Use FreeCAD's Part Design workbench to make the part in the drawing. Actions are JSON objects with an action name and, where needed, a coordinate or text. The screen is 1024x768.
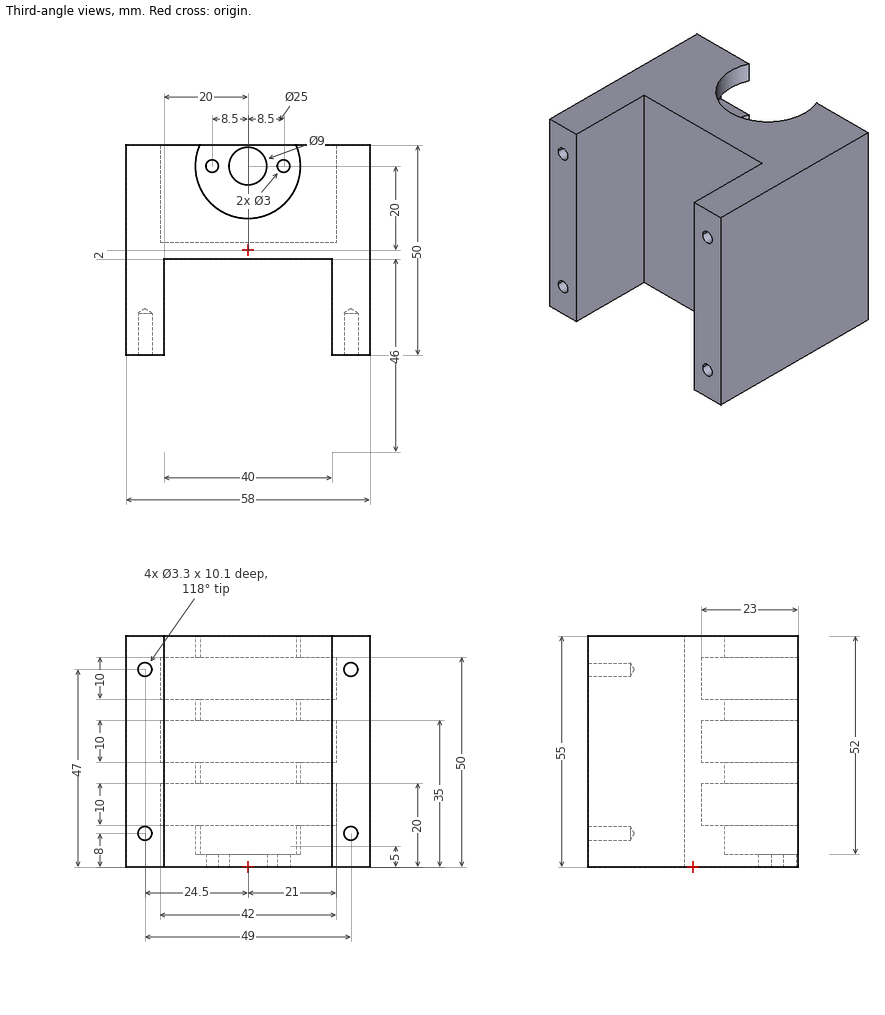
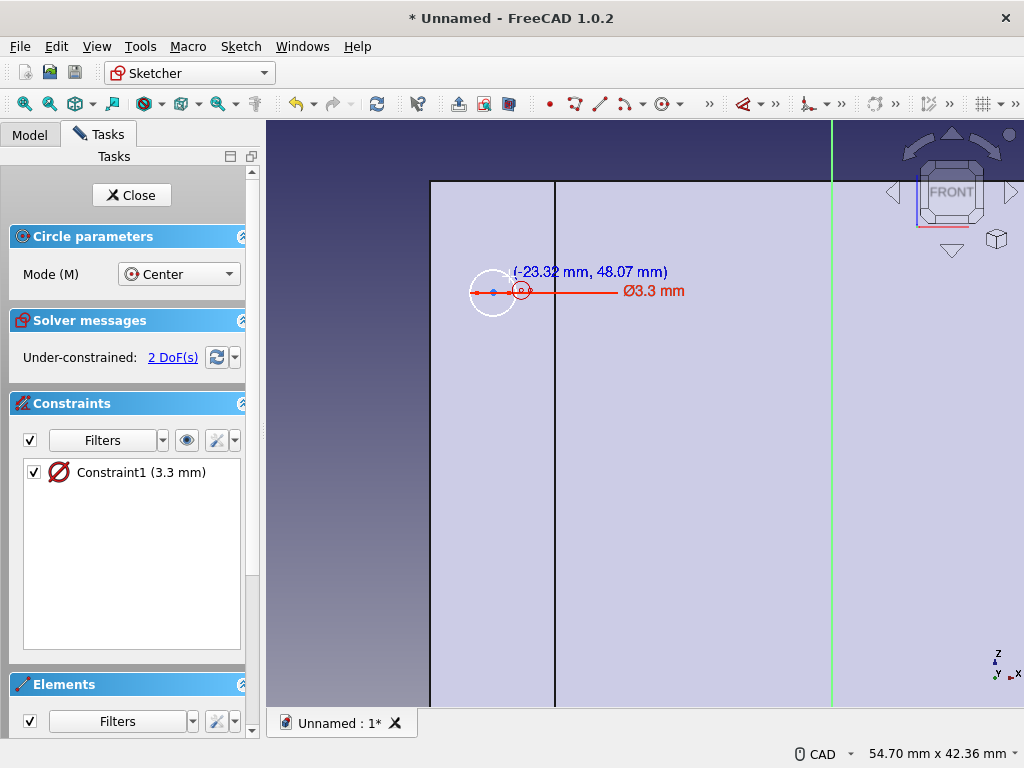
{"action": "scroll", "coordinate": [294, 179], "scroll_direction": "down", "scroll_amount": 3}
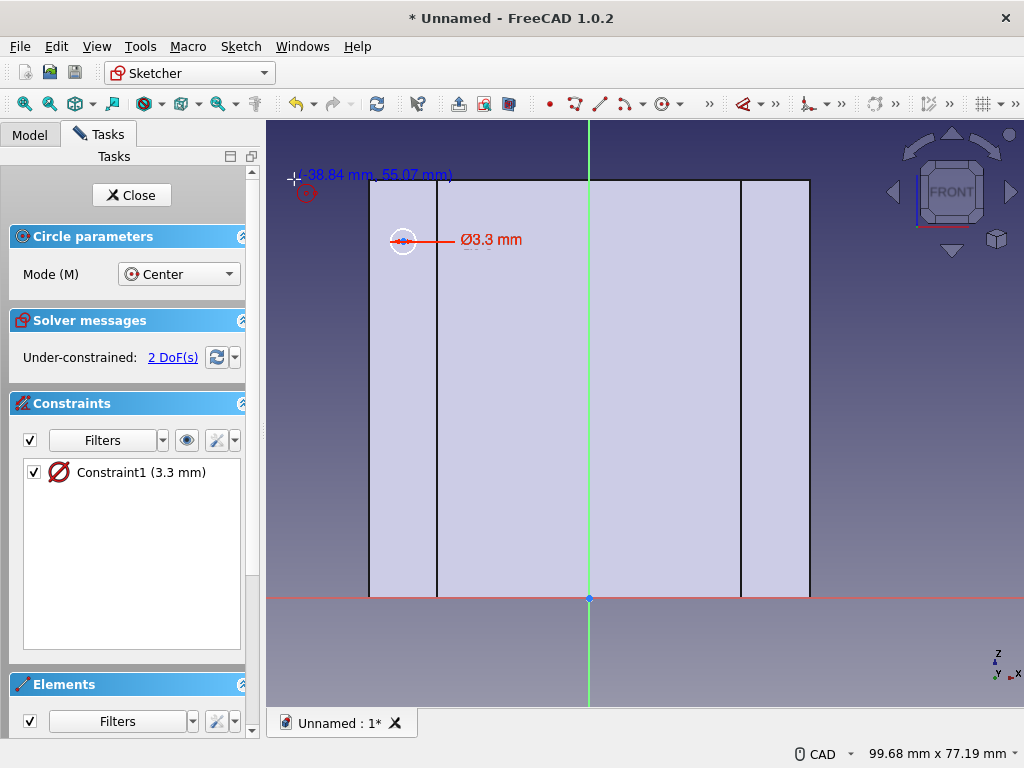
{"action": "scroll", "coordinate": [403, 538], "scroll_direction": "up", "scroll_amount": 3}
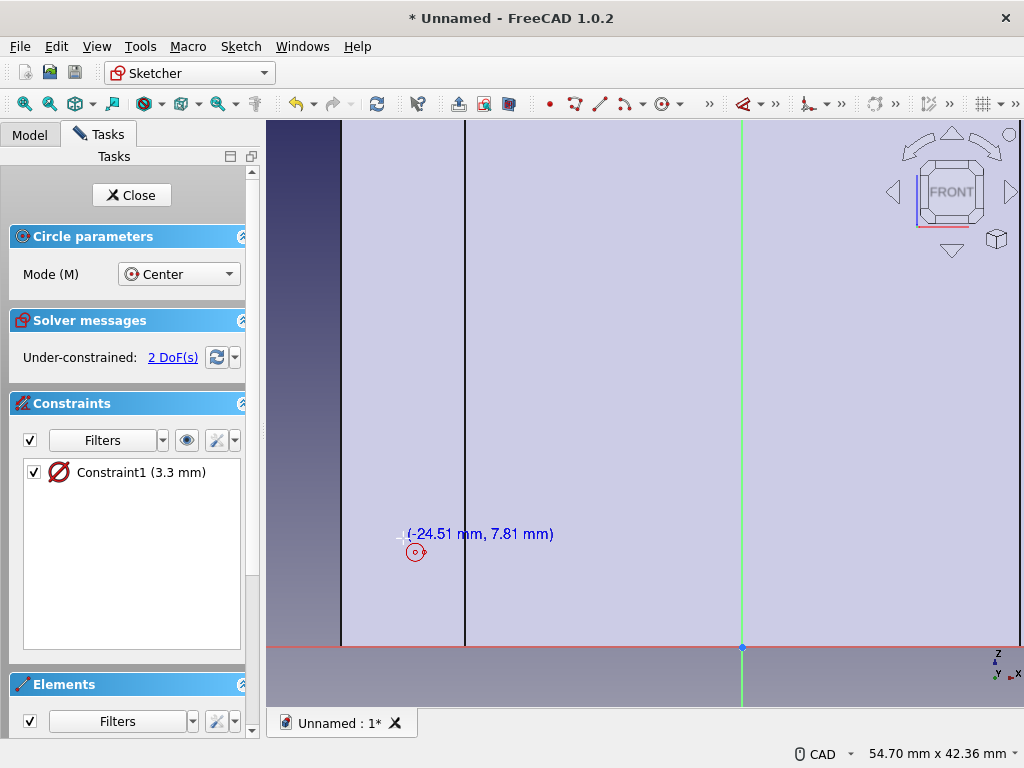
{"action": "left_click", "coordinate": [403, 537]}
{"action": "mouse_move", "coordinate": [419, 520]}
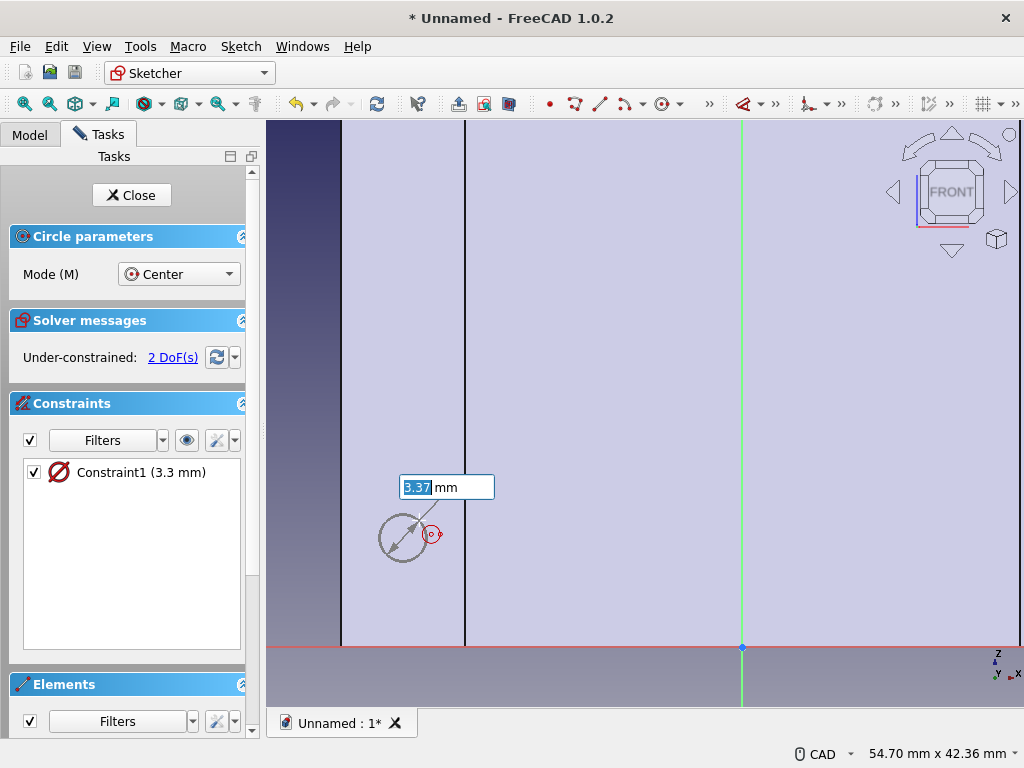
{"action": "type", "text": "3.3"}
{"action": "key", "text": "Return"}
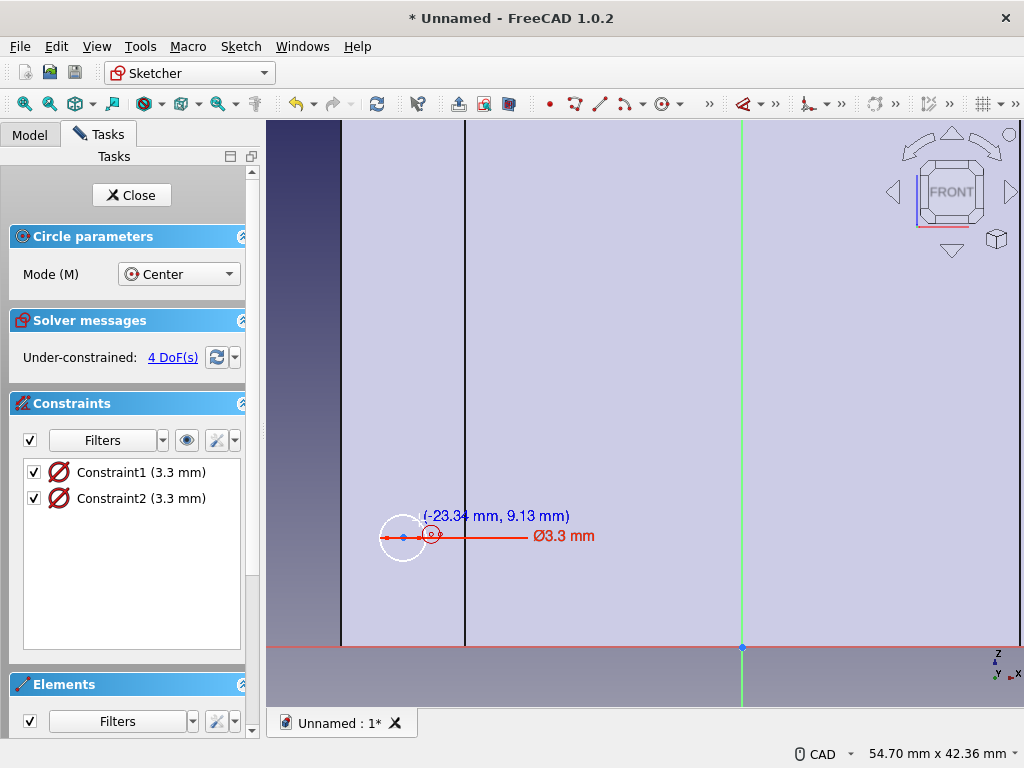
{"action": "scroll", "coordinate": [375, 539], "scroll_direction": "down", "scroll_amount": 3}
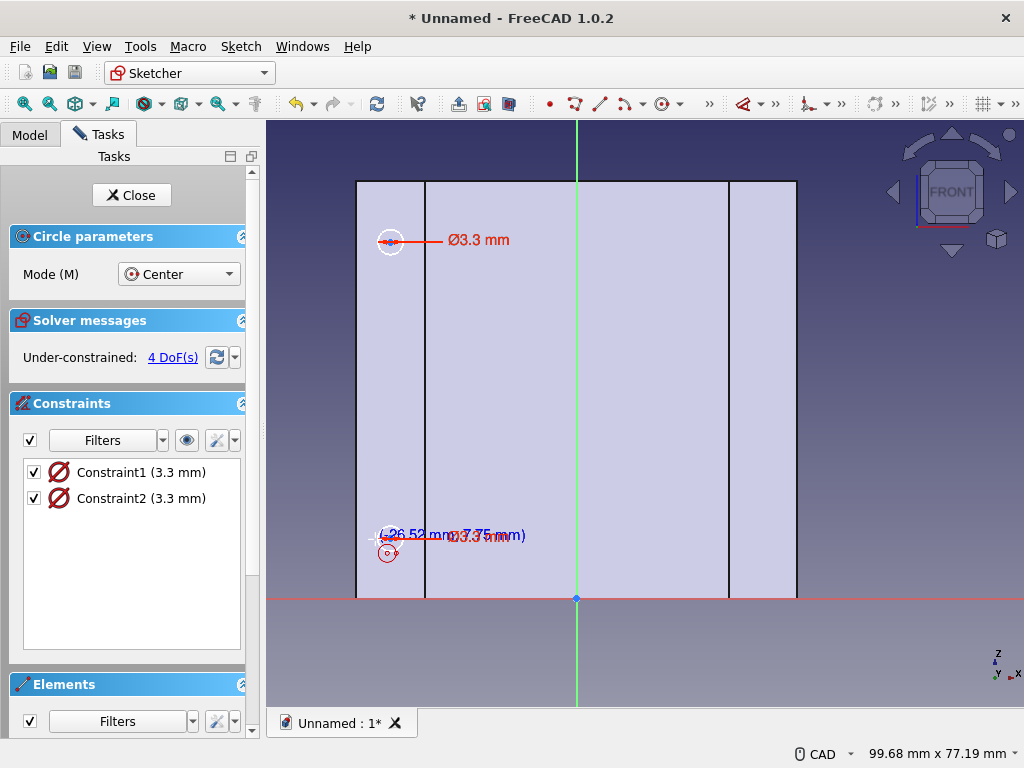
{"action": "scroll", "coordinate": [763, 538], "scroll_direction": "up", "scroll_amount": 3}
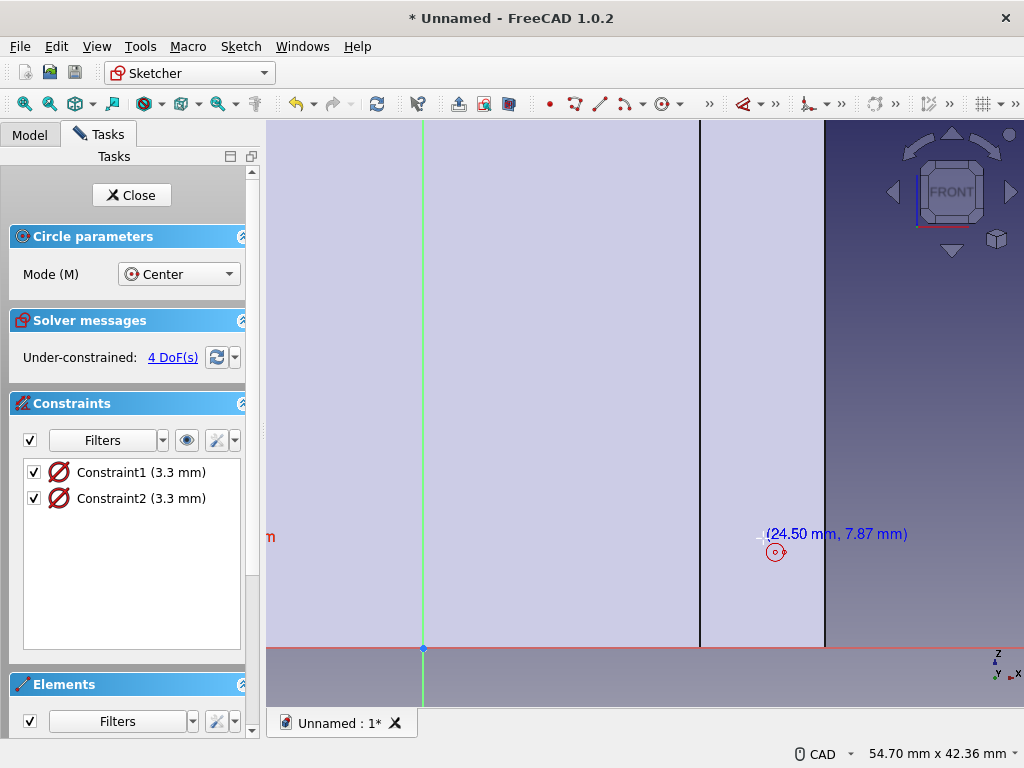
{"action": "left_click", "coordinate": [762, 537]}
{"action": "mouse_move", "coordinate": [779, 521]}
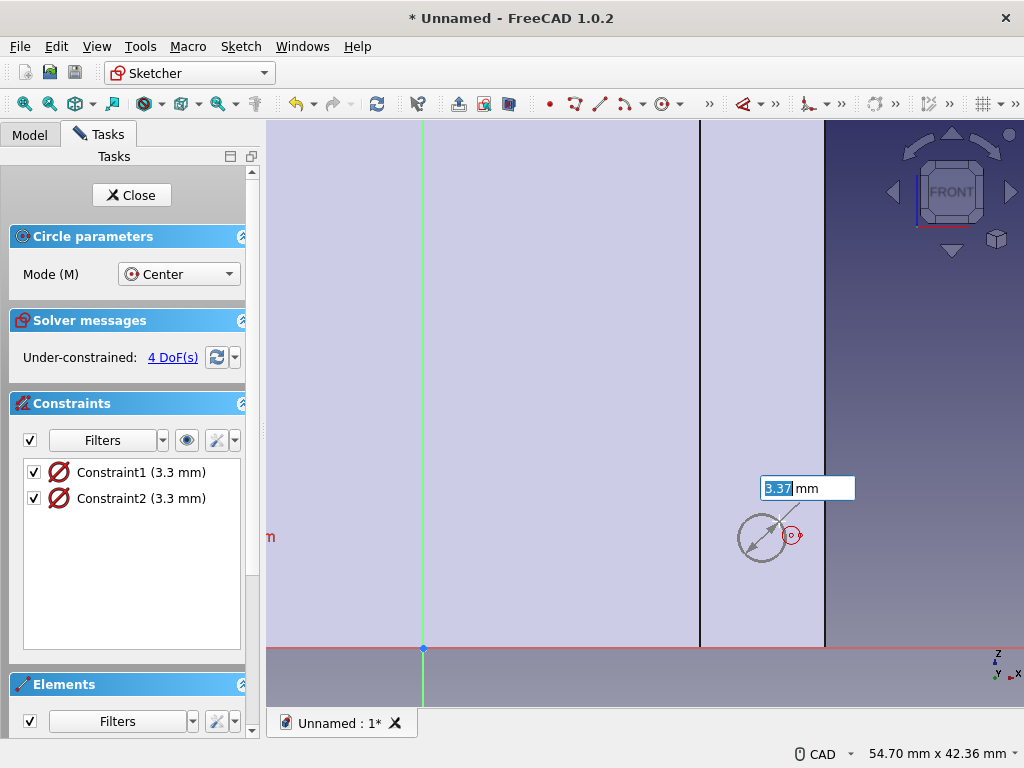
{"action": "type", "text": "3.3"}
{"action": "key", "text": "Return"}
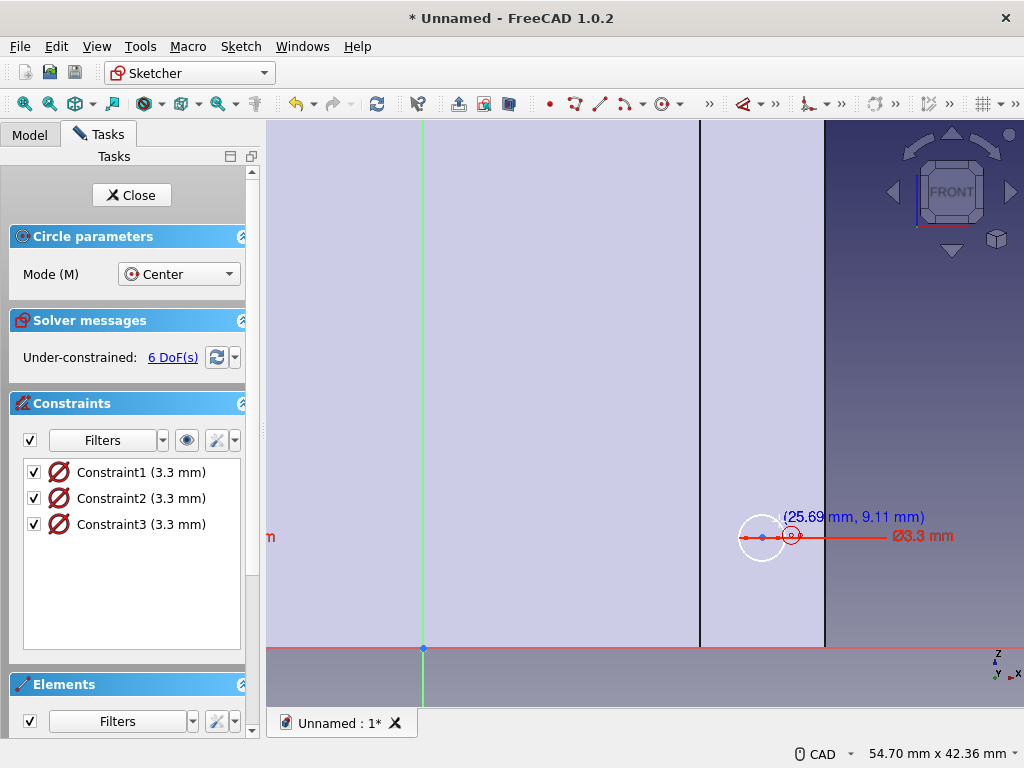
{"action": "scroll", "coordinate": [763, 538], "scroll_direction": "down", "scroll_amount": 3}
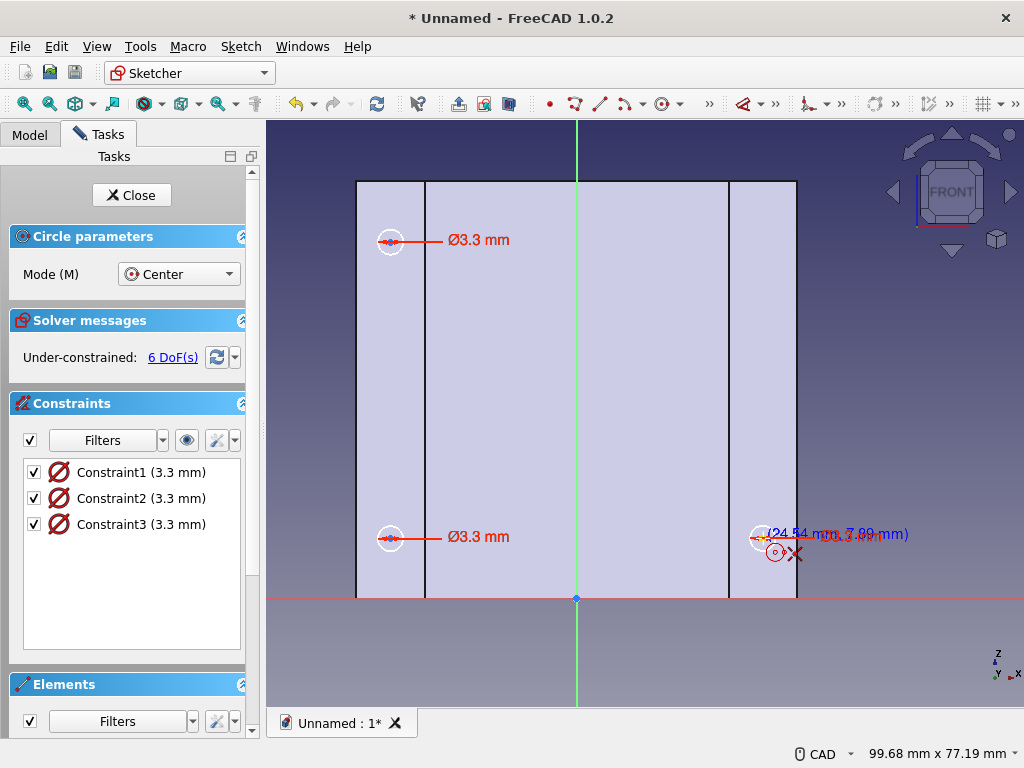
{"action": "scroll", "coordinate": [763, 241], "scroll_direction": "up", "scroll_amount": 3}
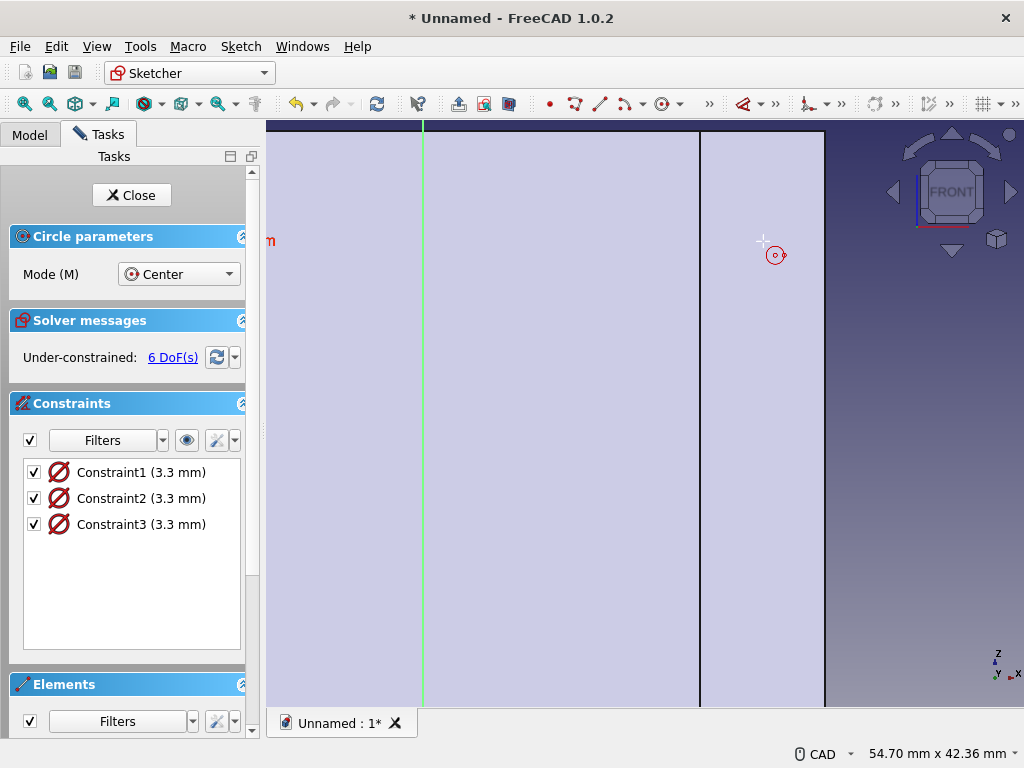
{"action": "left_click", "coordinate": [762, 242]}
{"action": "mouse_move", "coordinate": [779, 225]}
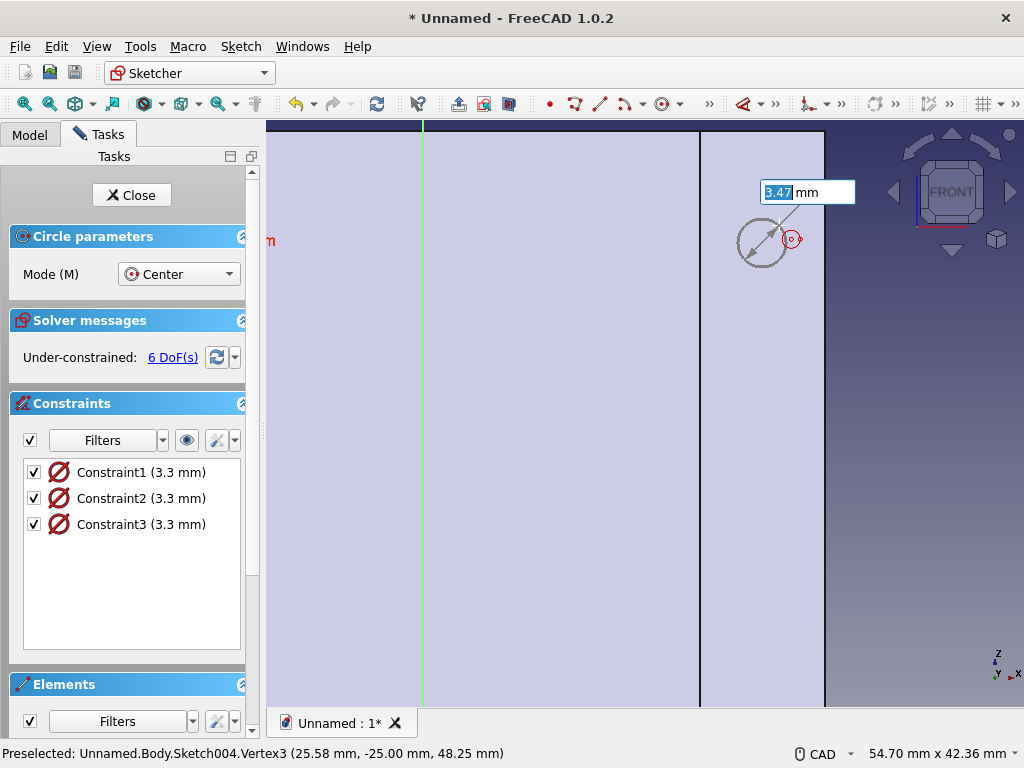
{"action": "type", "text": "3.3"}
{"action": "key", "text": "Return"}
{"action": "key", "text": "Escape"}